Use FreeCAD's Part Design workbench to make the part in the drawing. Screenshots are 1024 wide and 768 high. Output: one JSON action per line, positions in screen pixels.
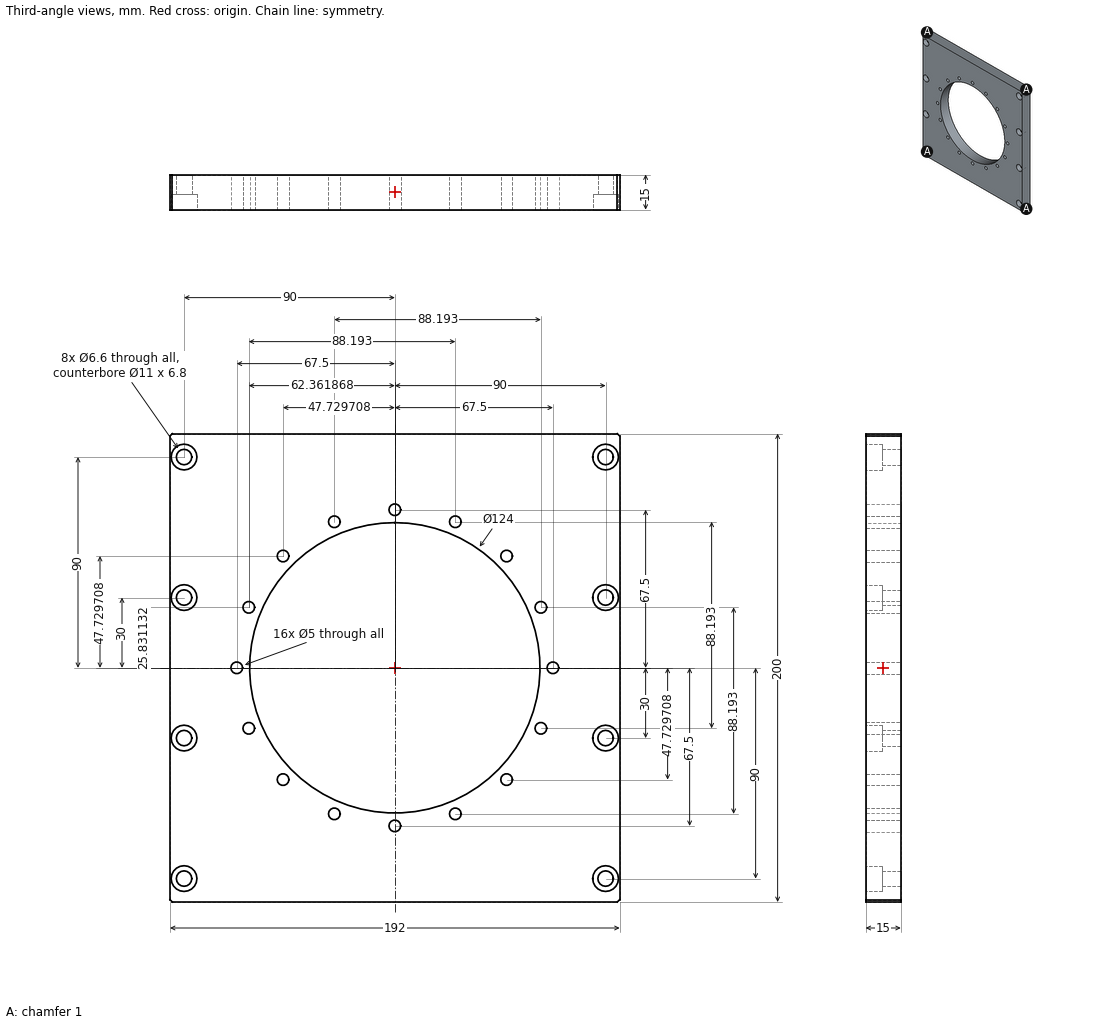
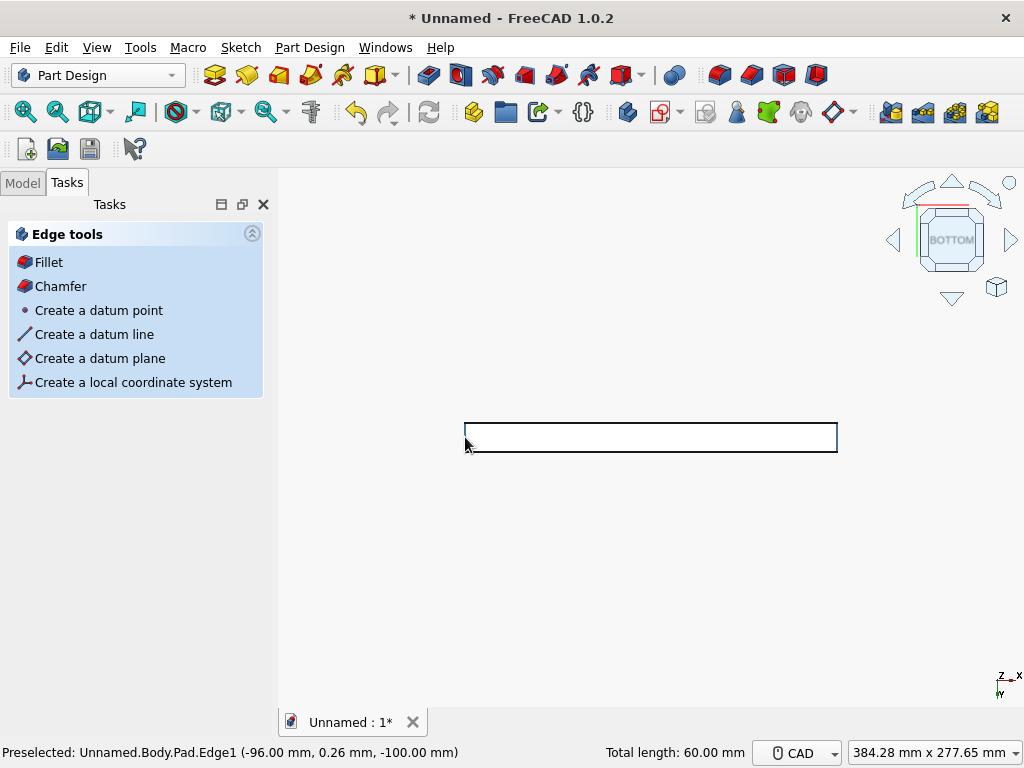
{"action": "left_click", "coordinate": [752, 76]}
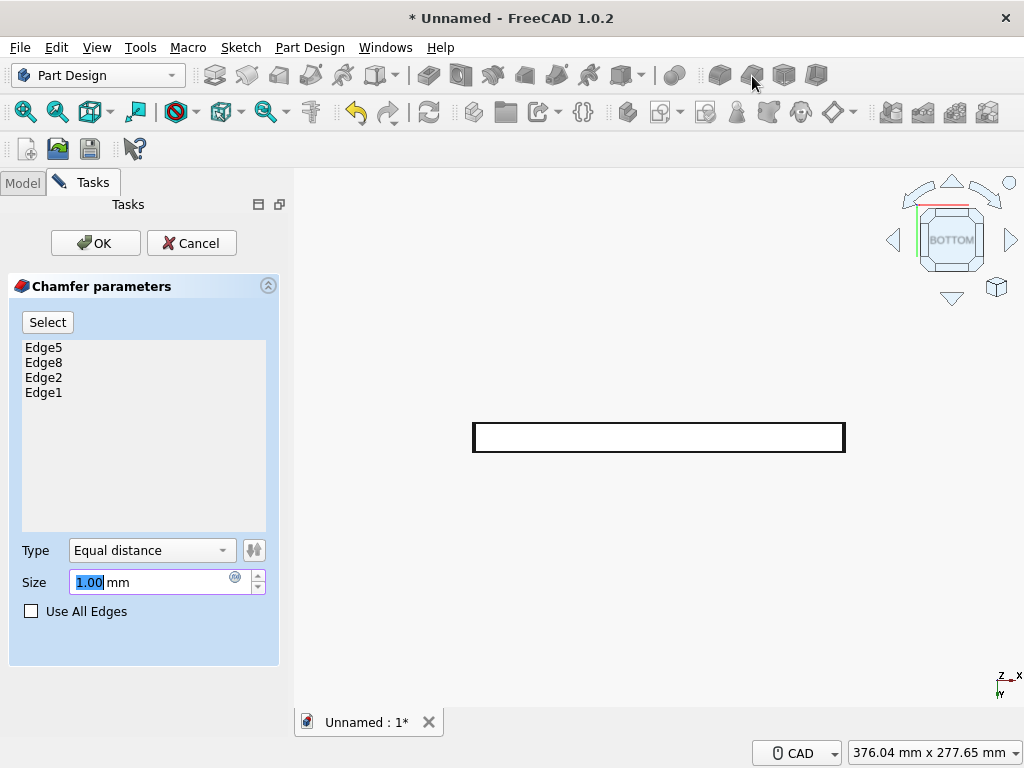
{"action": "type", "text": "1"}
{"action": "key", "text": "Tab"}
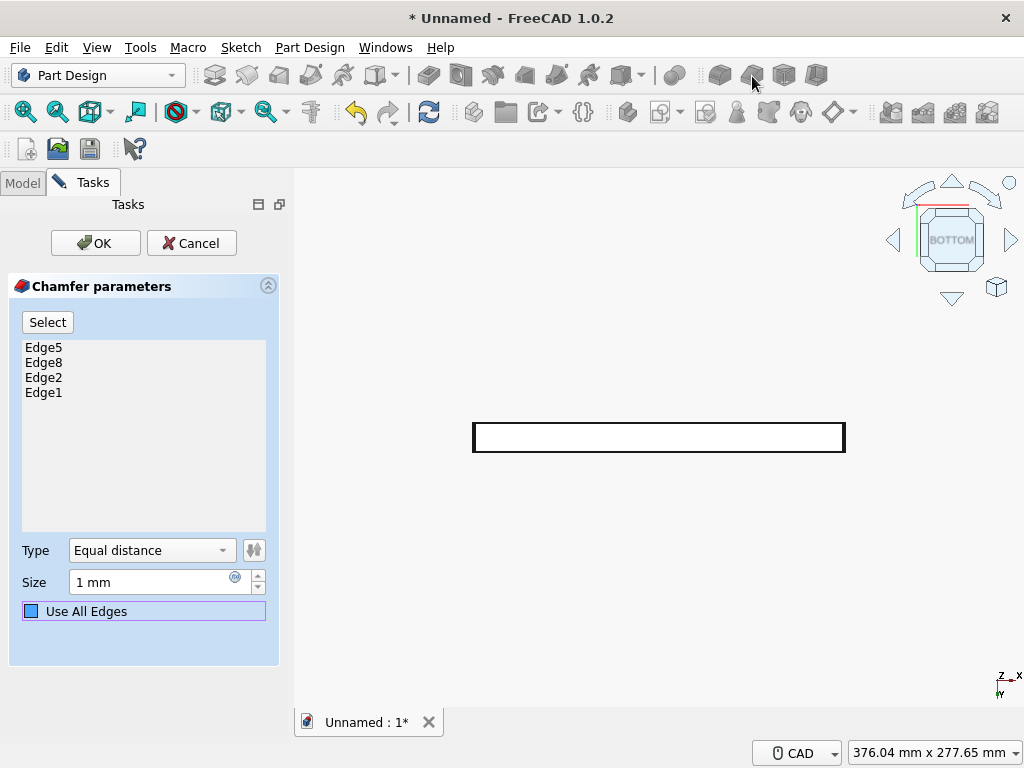
{"action": "left_click", "coordinate": [96, 243]}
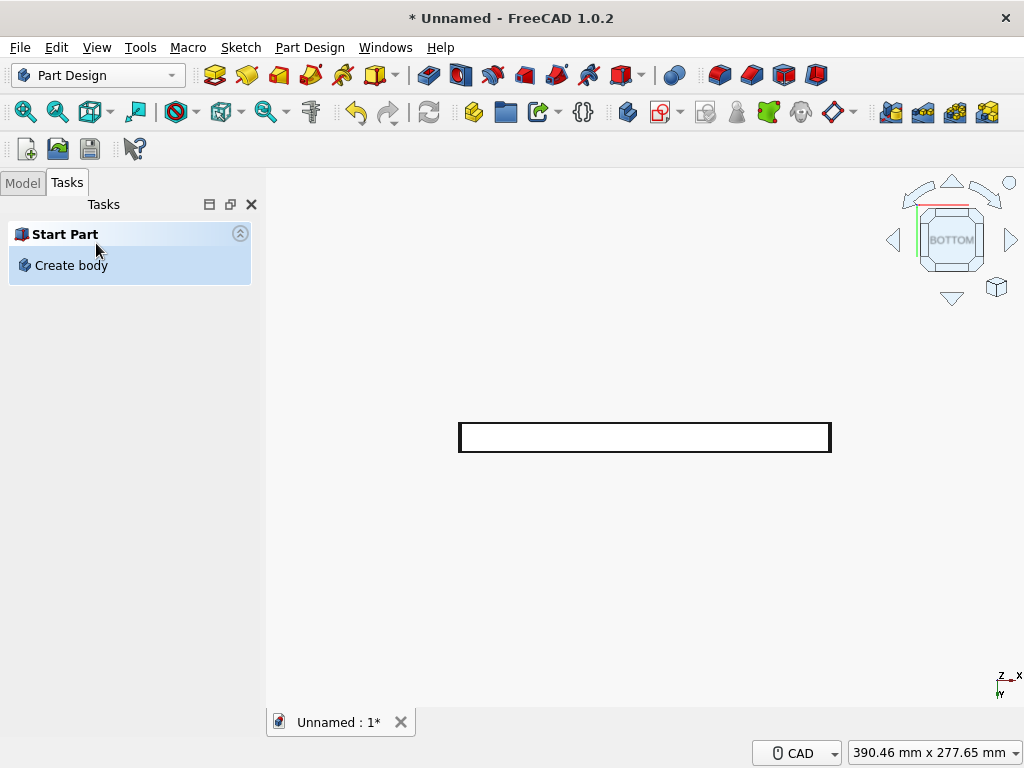
{"action": "key", "text": "0"}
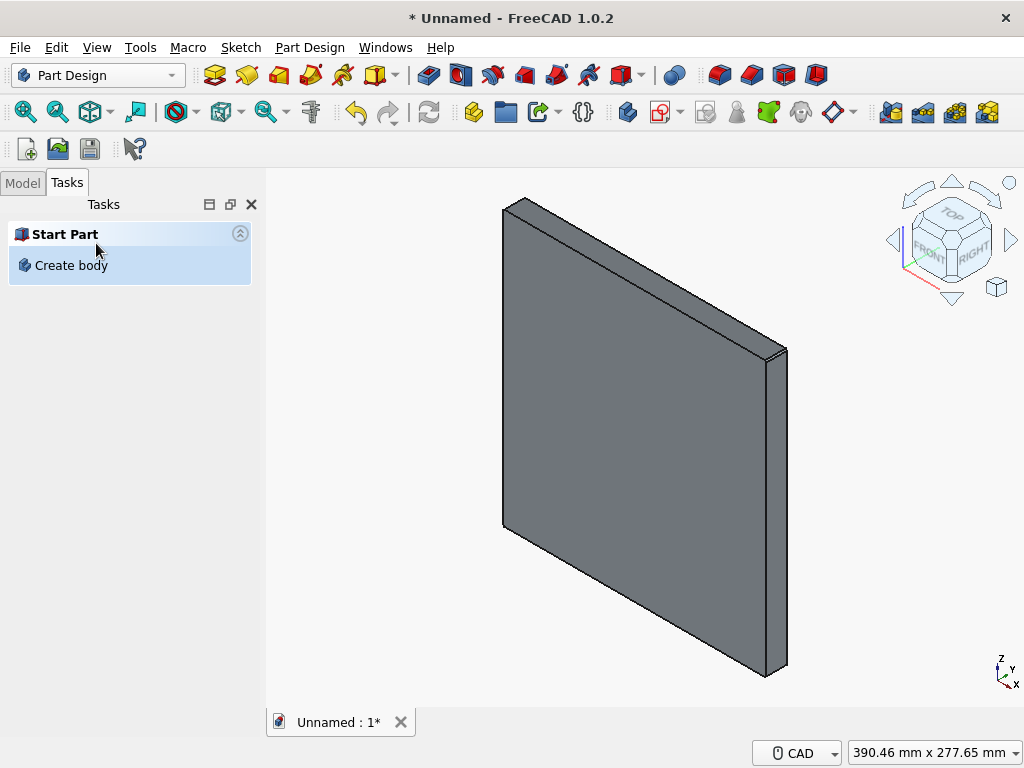
{"action": "left_click", "coordinate": [635, 442]}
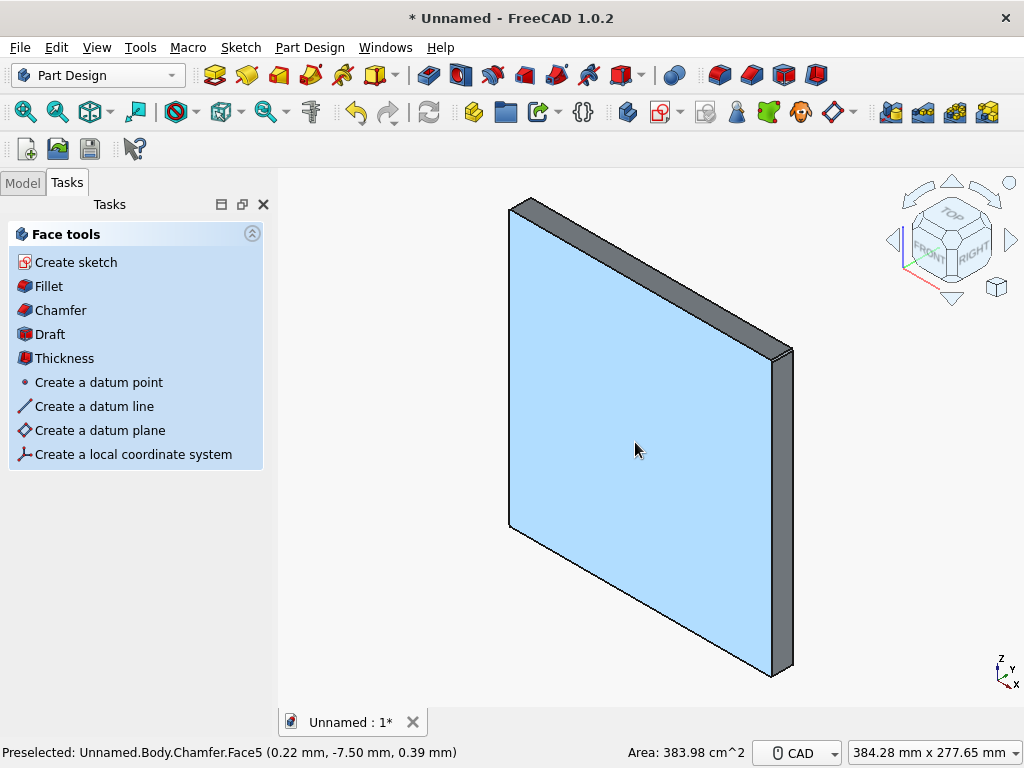
{"action": "left_click", "coordinate": [660, 112]}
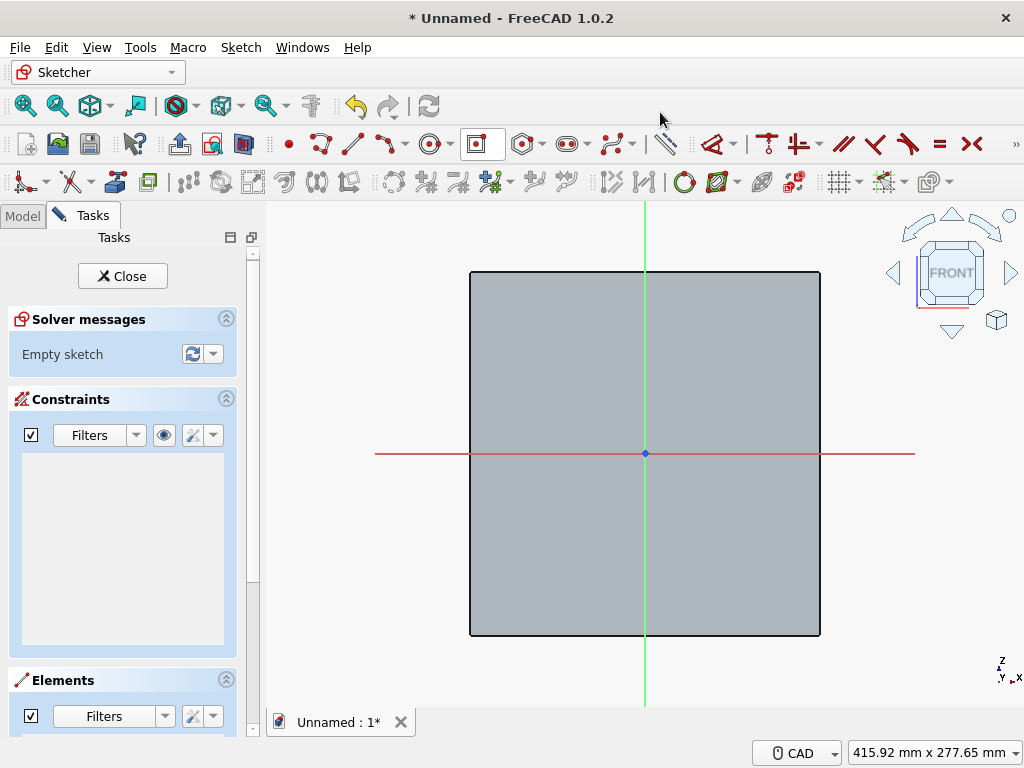
{"action": "left_click", "coordinate": [430, 144]}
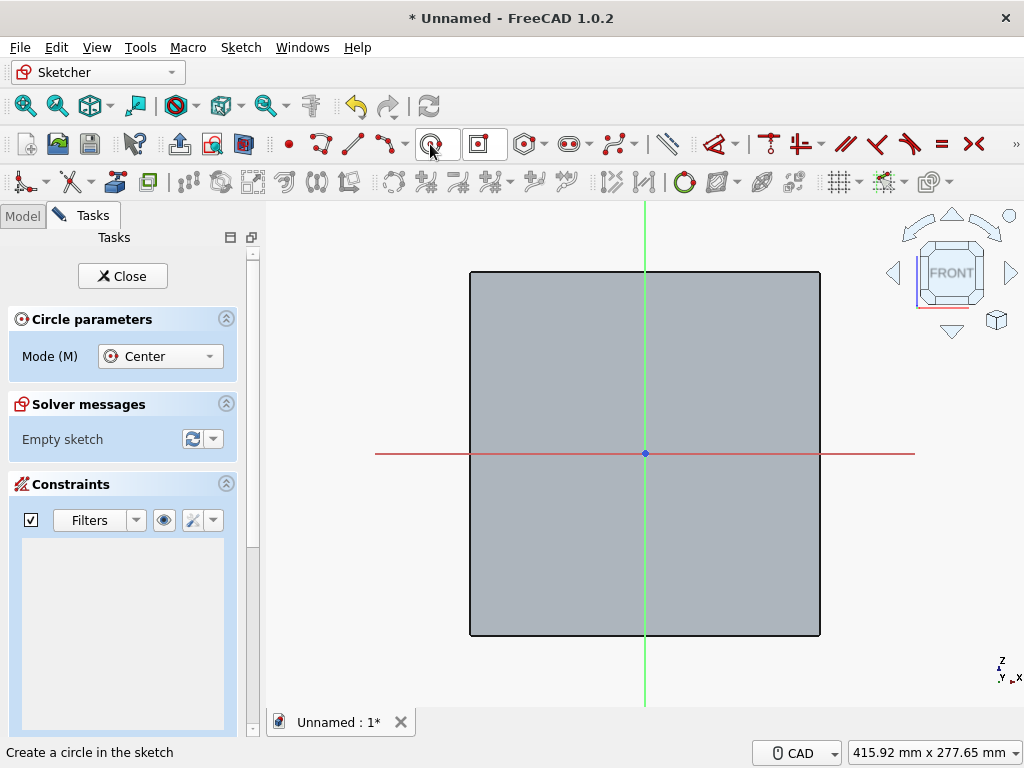
{"action": "scroll", "coordinate": [481, 290], "scroll_direction": "up", "scroll_amount": 7}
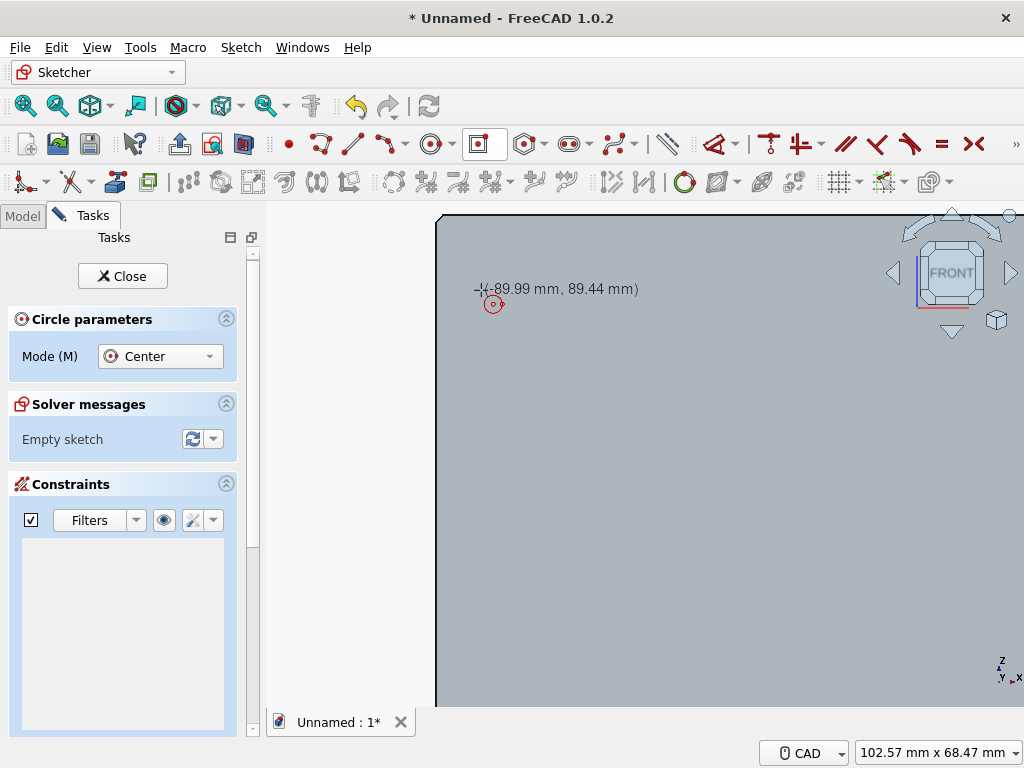
{"action": "scroll", "coordinate": [390, 290], "scroll_direction": "down", "scroll_amount": 7}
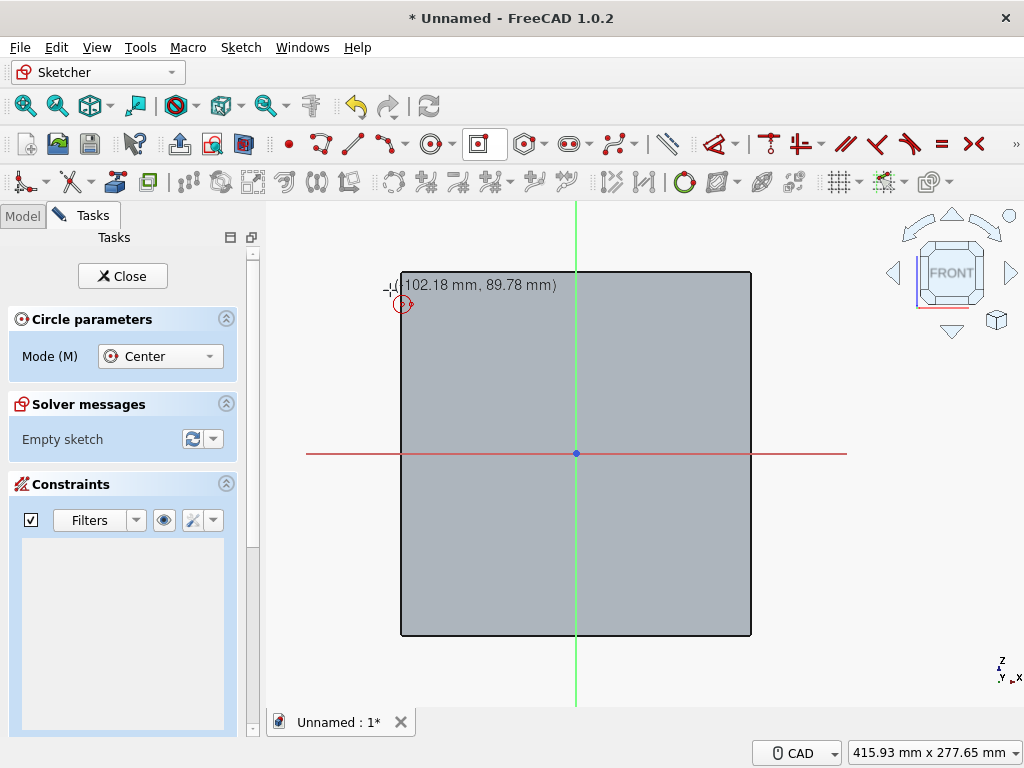
{"action": "left_click", "coordinate": [412, 290]}
{"action": "mouse_move", "coordinate": [417, 286]}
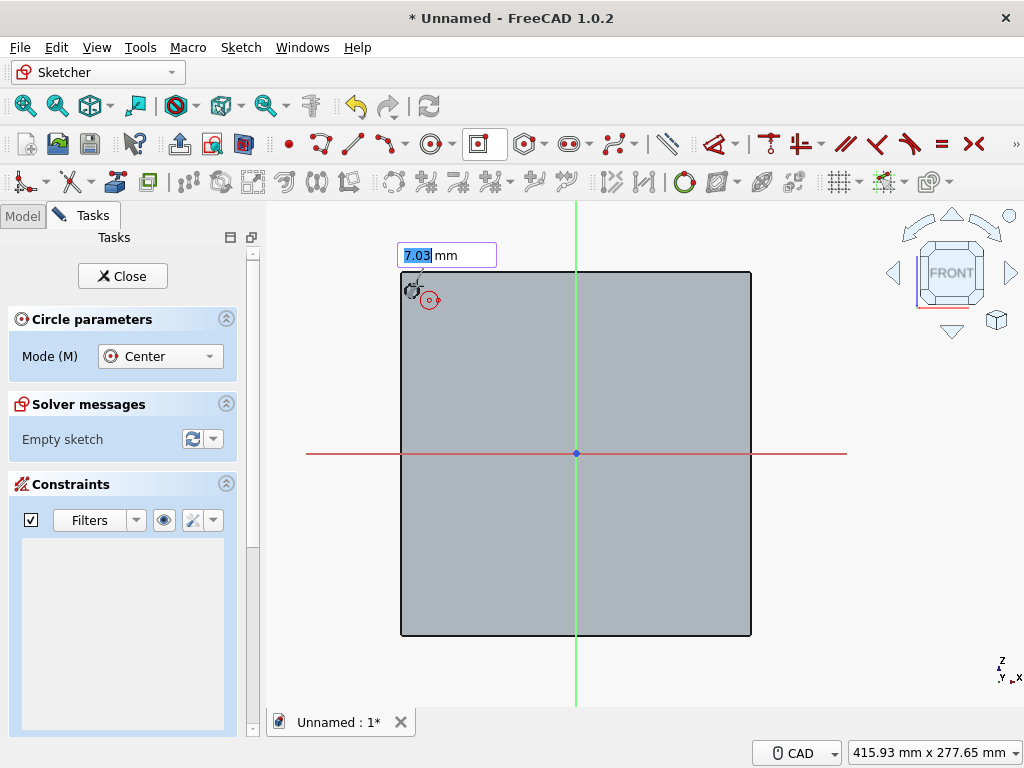
{"action": "type", "text": "6.6"}
{"action": "key", "text": "Return"}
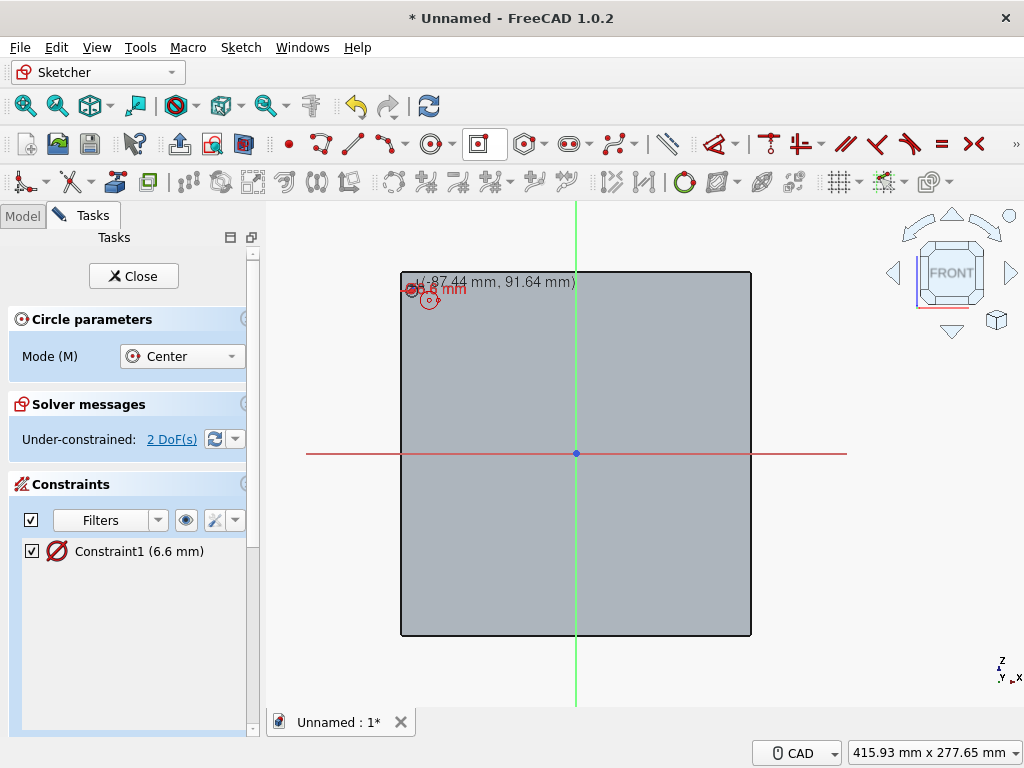
{"action": "scroll", "coordinate": [412, 399], "scroll_direction": "up", "scroll_amount": 7}